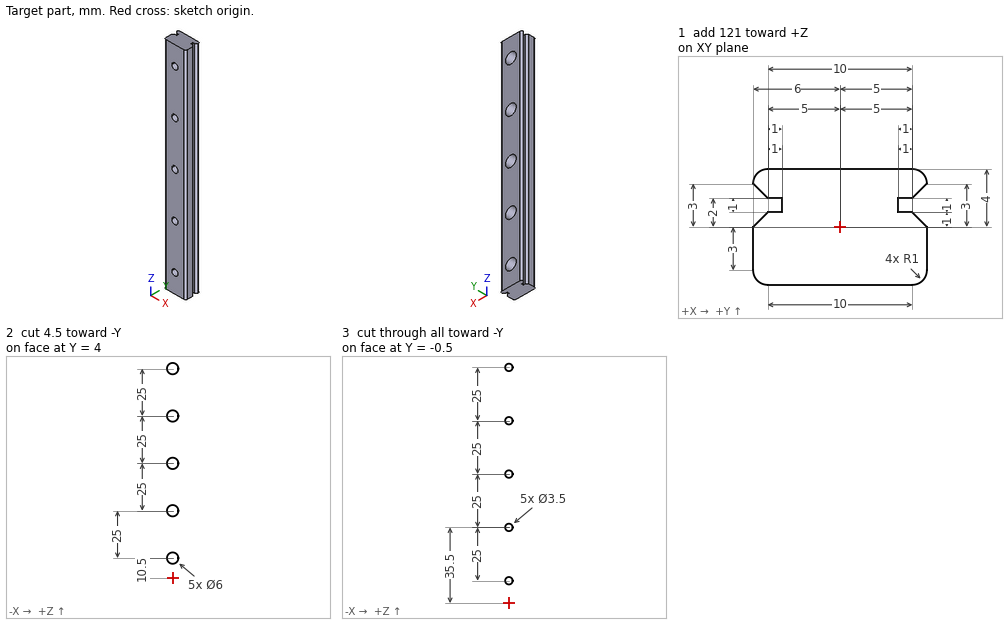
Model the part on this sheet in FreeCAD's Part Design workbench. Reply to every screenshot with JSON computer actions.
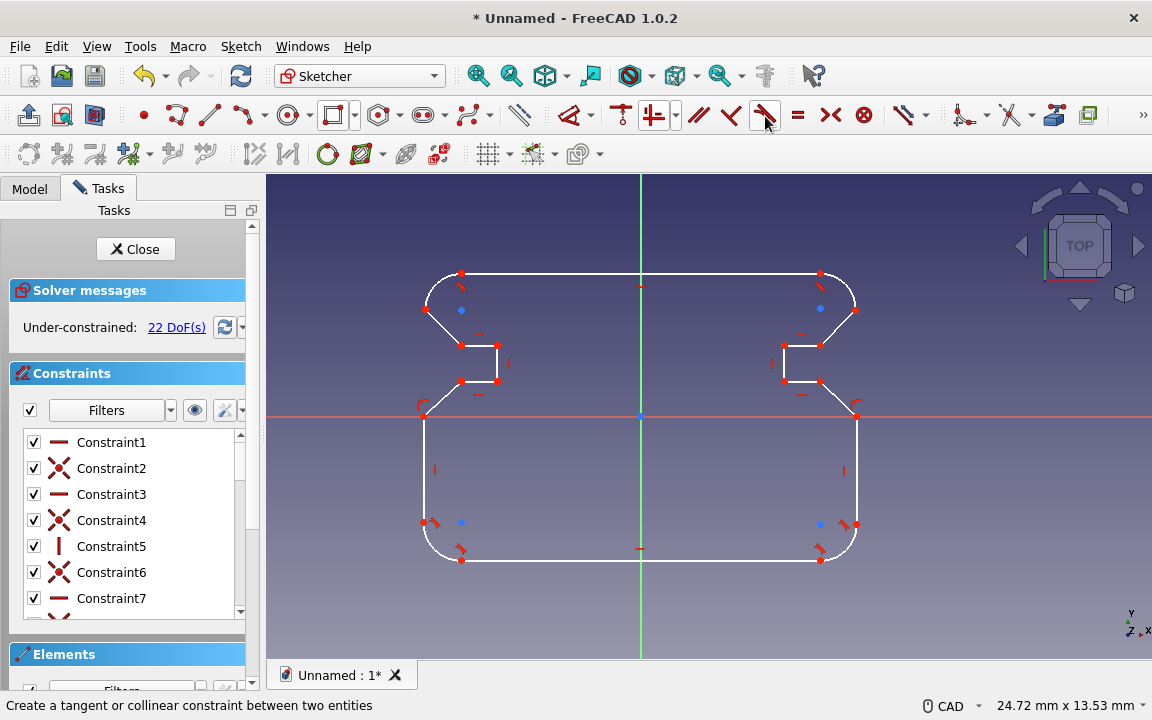
{"action": "left_click", "coordinate": [445, 278]}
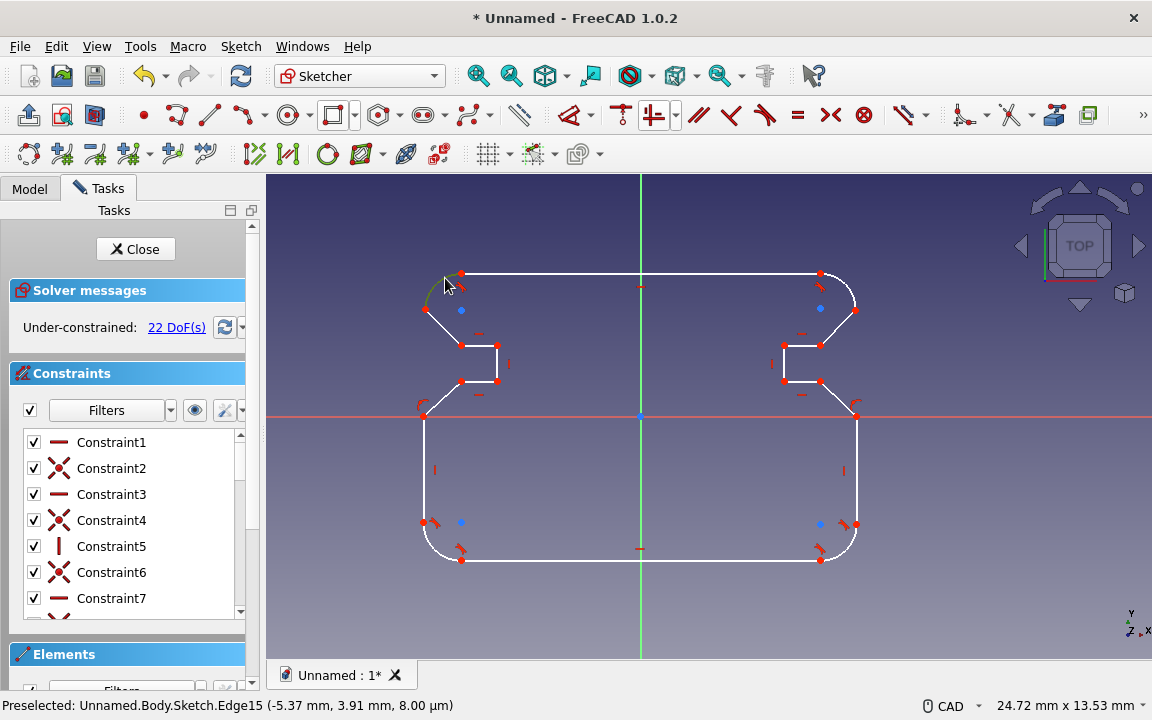
{"action": "left_click", "coordinate": [428, 540]}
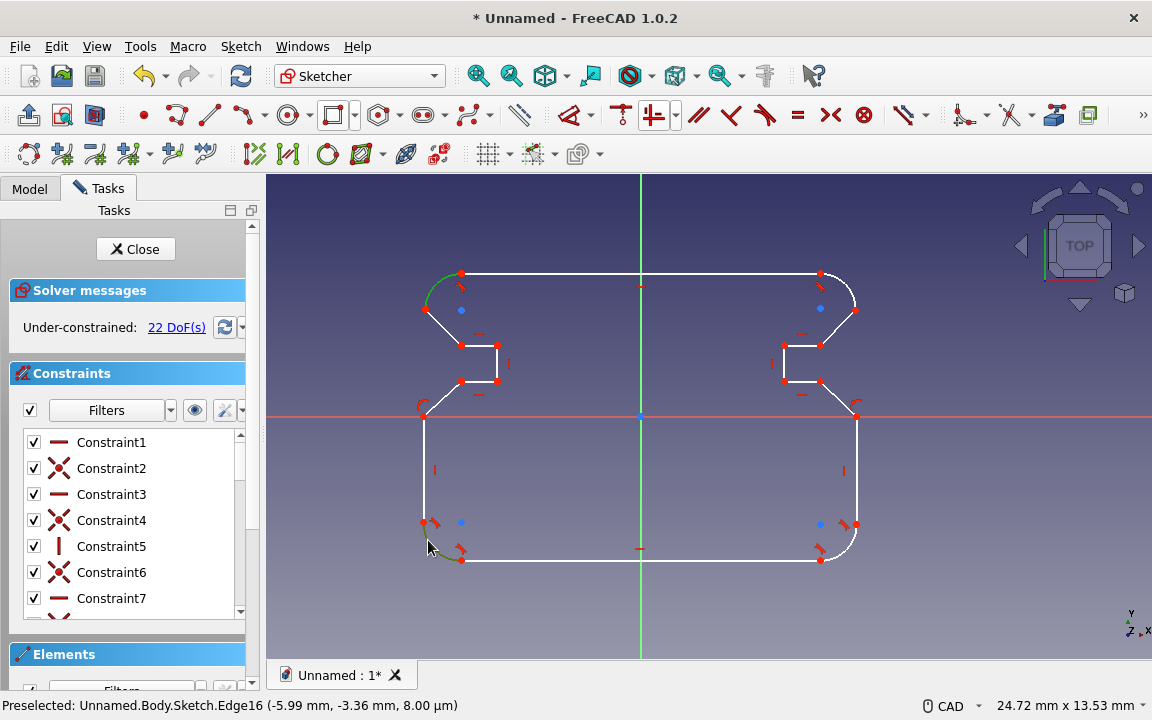
{"action": "left_click", "coordinate": [837, 557]}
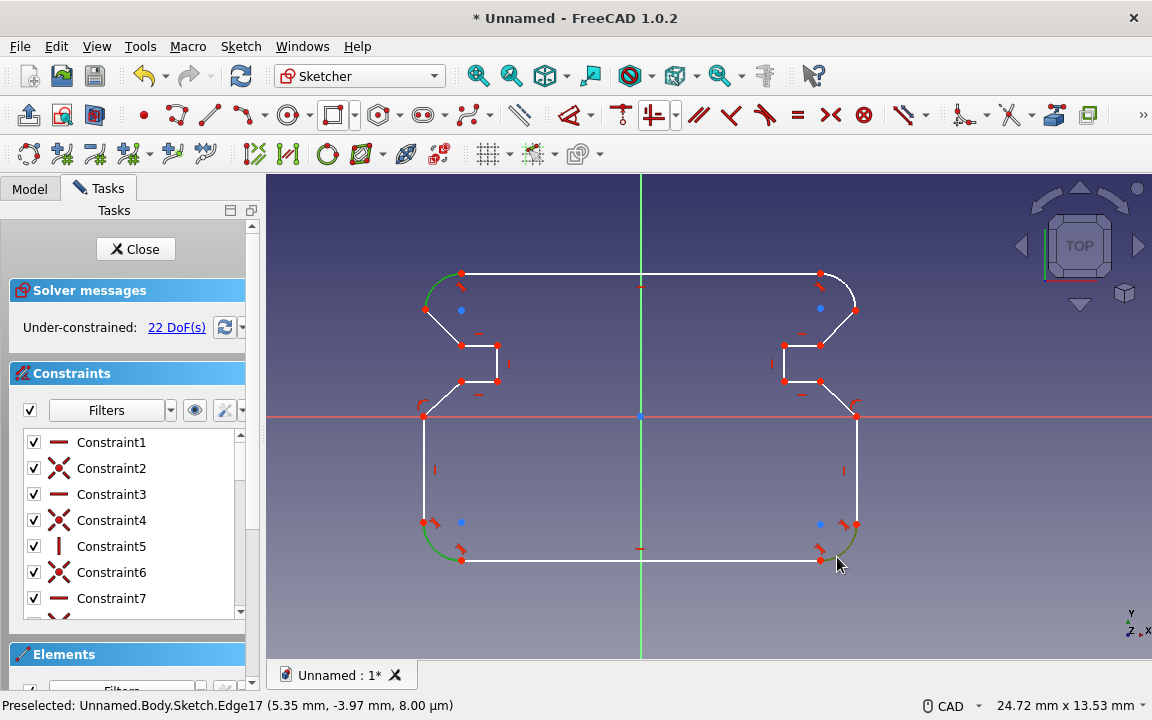
{"action": "left_click", "coordinate": [852, 294]}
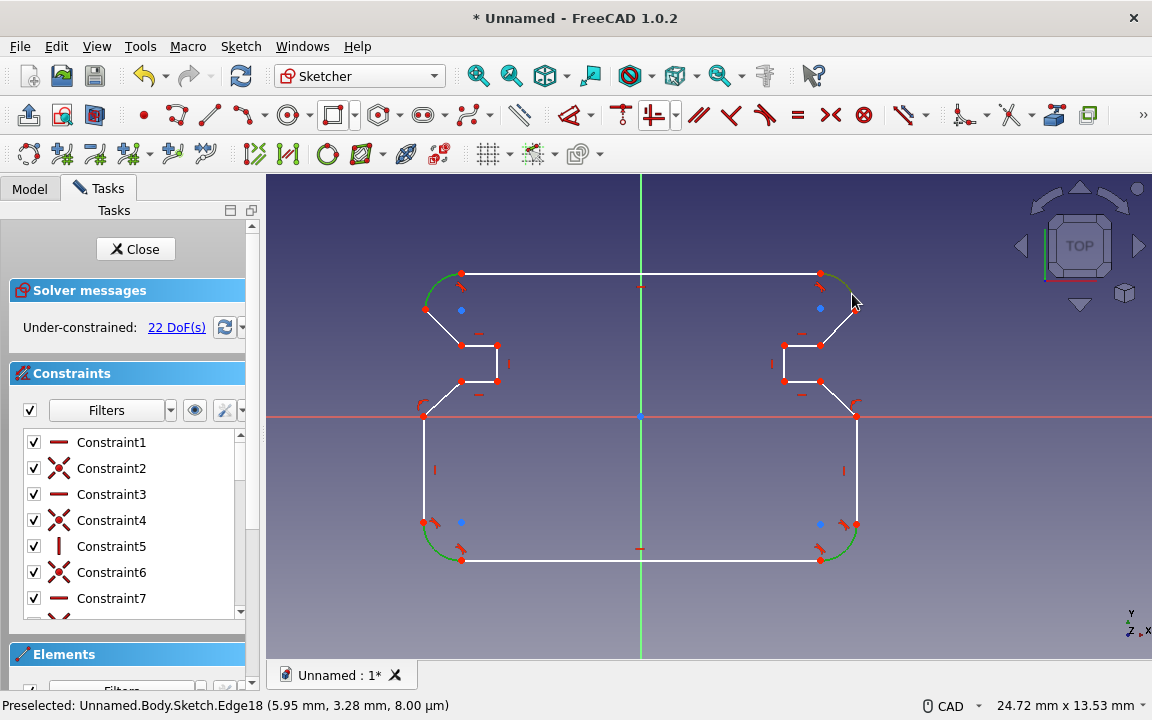
{"action": "left_click", "coordinate": [798, 116]}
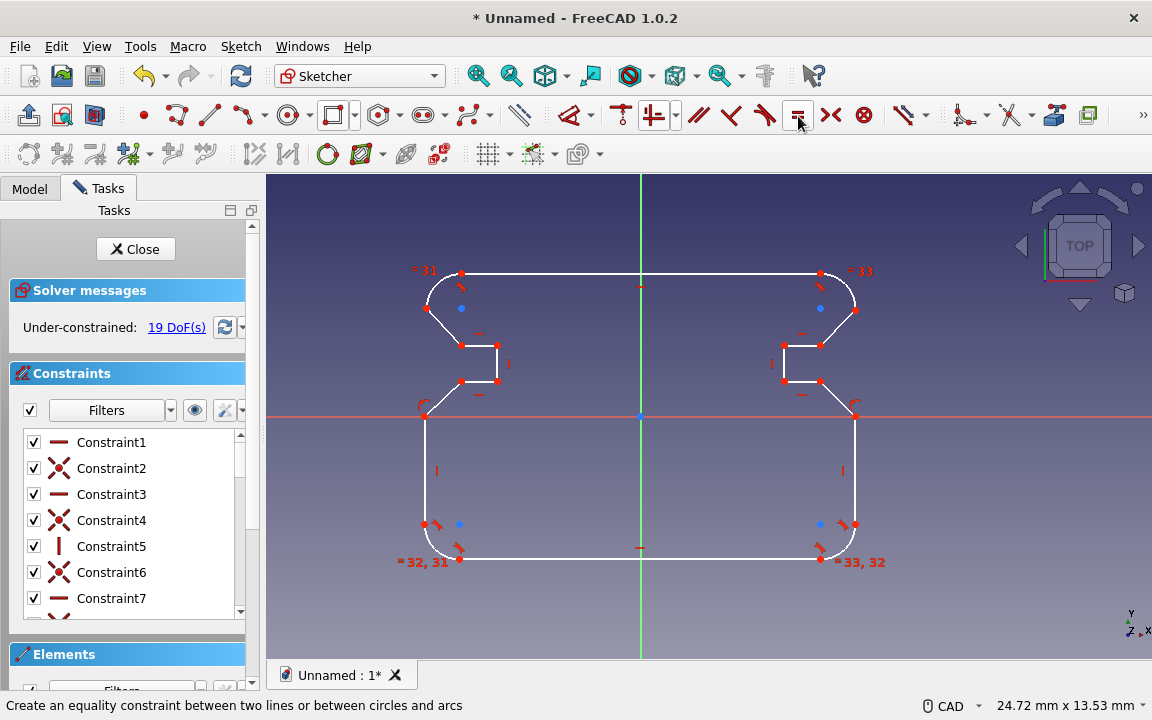
{"action": "left_click", "coordinate": [568, 116]}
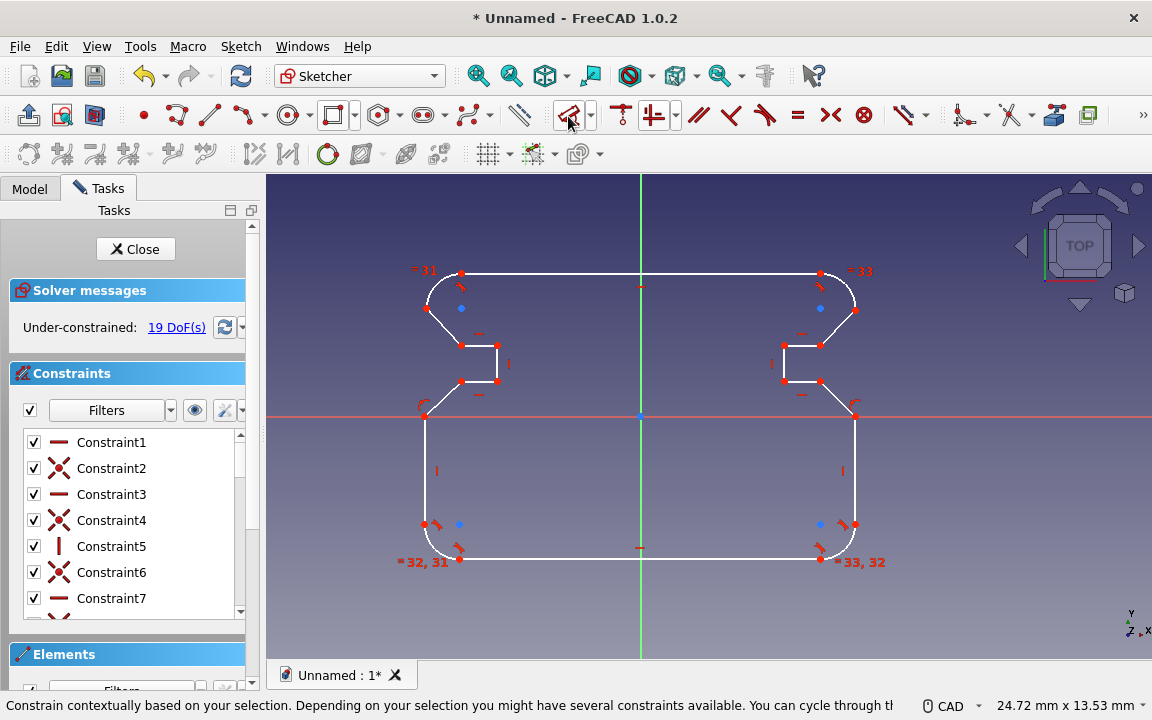
{"action": "left_click", "coordinate": [446, 278]}
{"action": "left_click", "coordinate": [432, 249]}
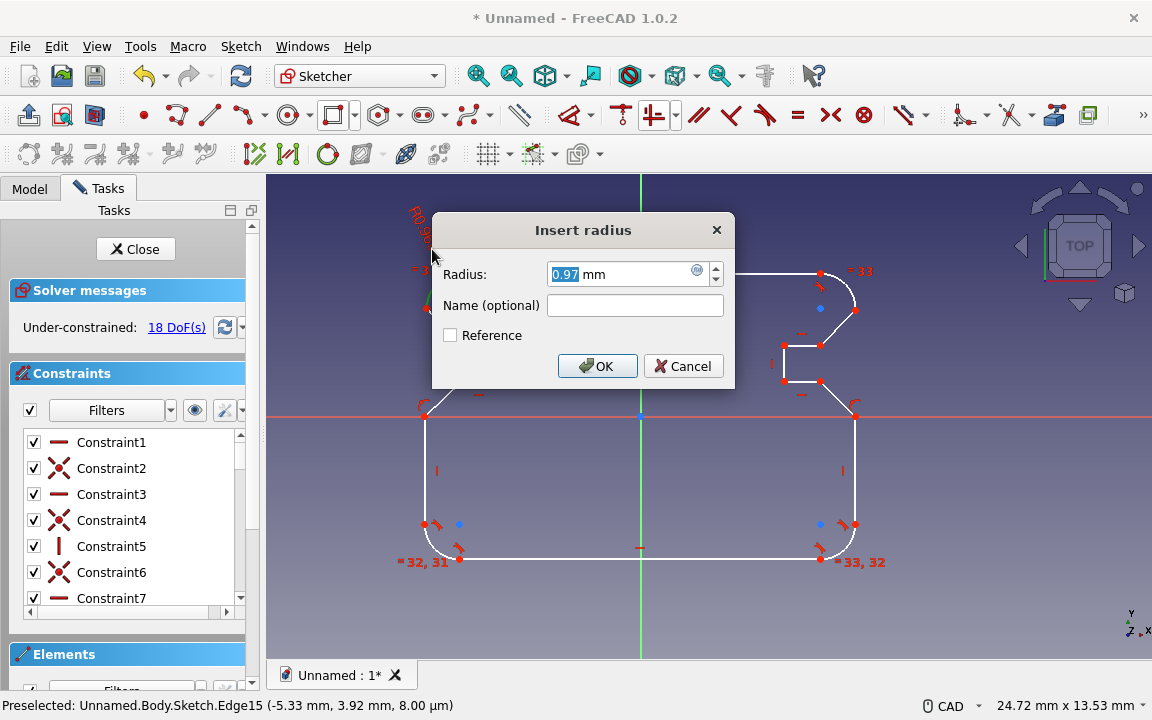
{"action": "type", "text": "1"}
{"action": "key", "text": "Return"}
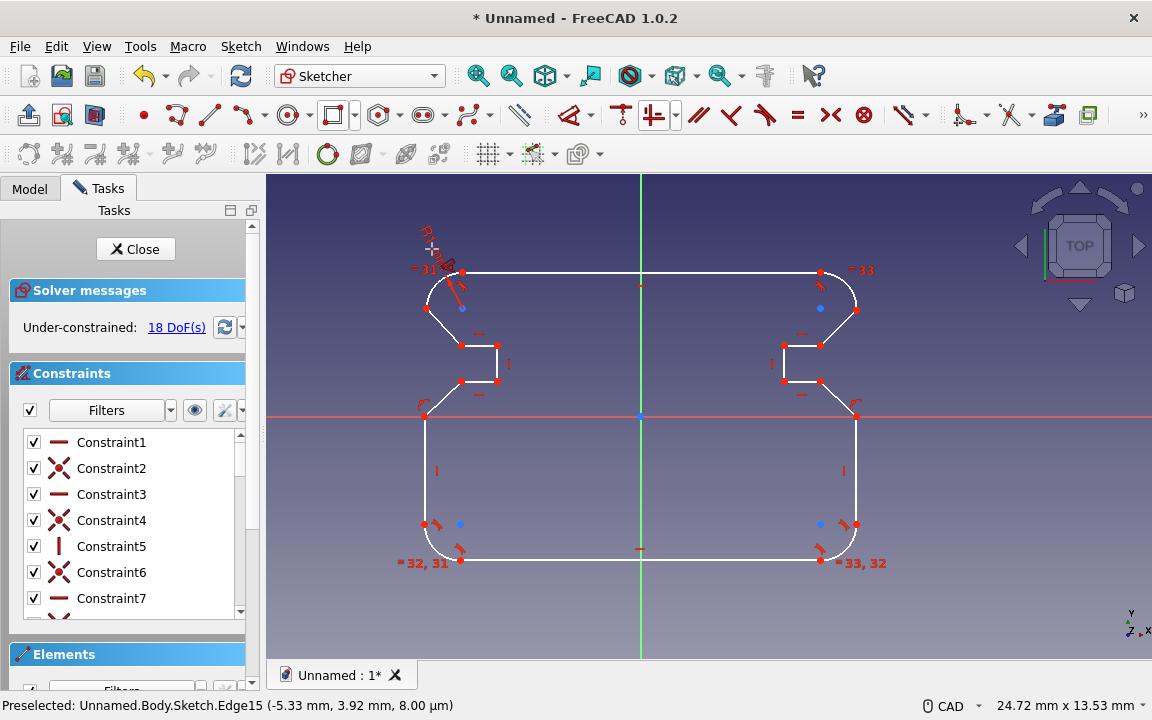
{"action": "scroll", "coordinate": [472, 346], "scroll_direction": "up", "scroll_amount": 2}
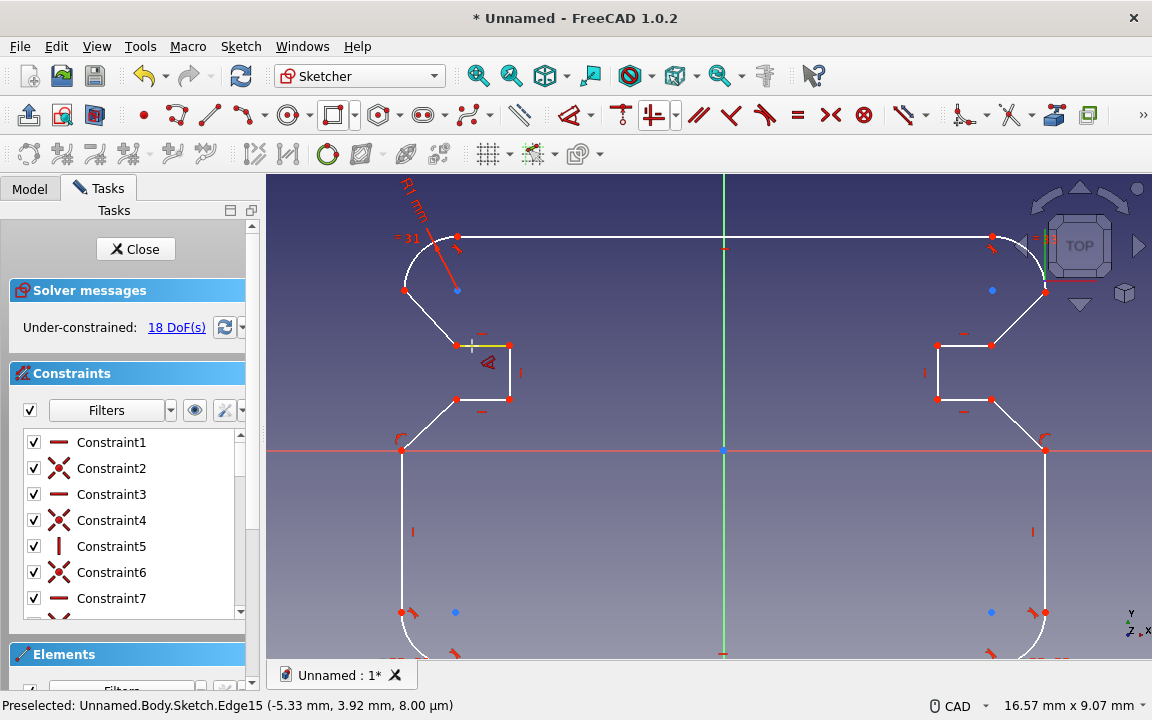
{"action": "left_click", "coordinate": [472, 346]}
{"action": "left_click", "coordinate": [483, 312]}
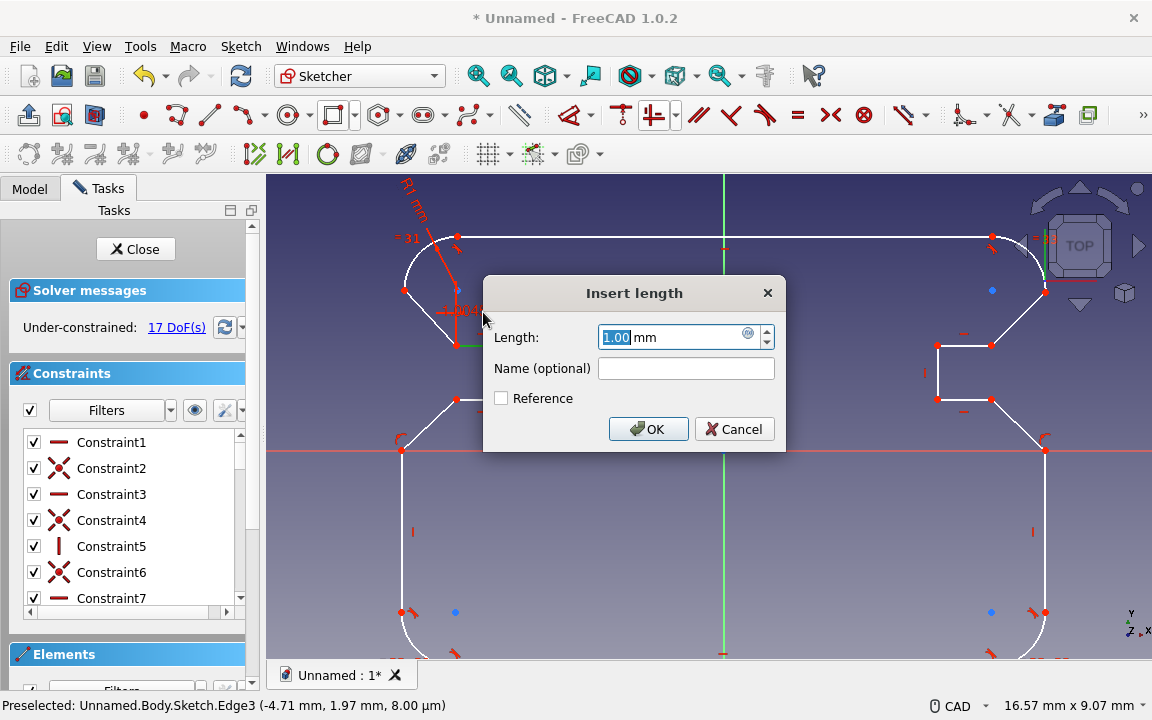
{"action": "type", "text": "1"}
{"action": "key", "text": "Return"}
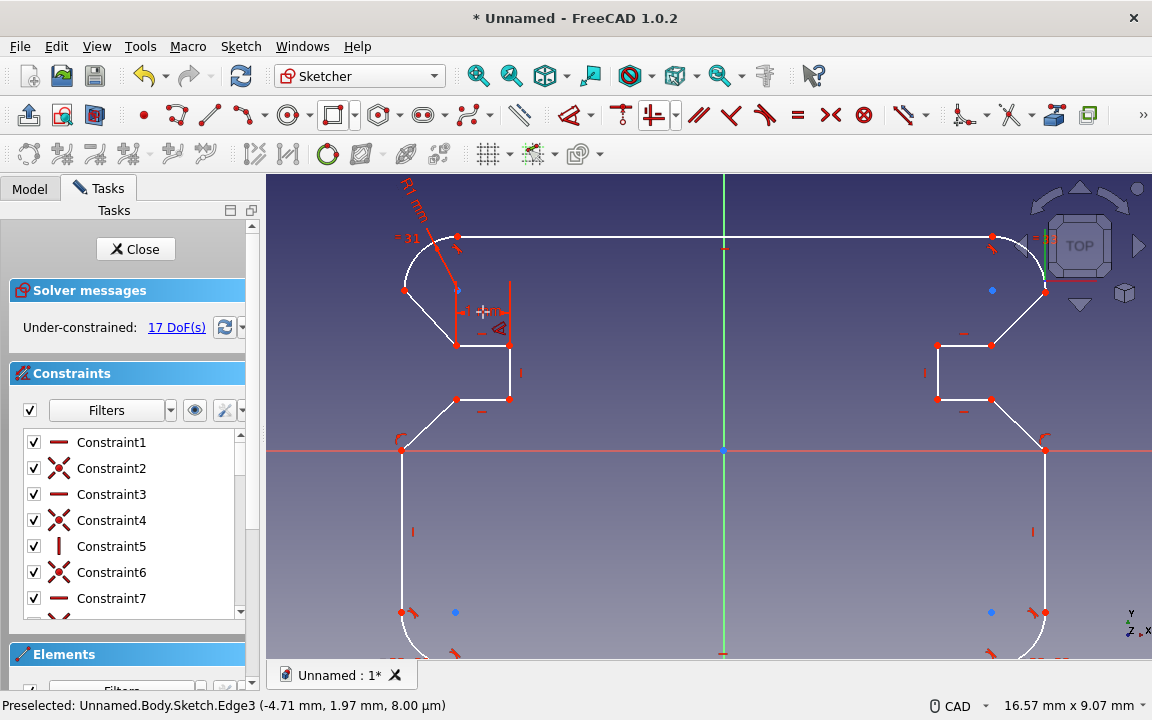
{"action": "left_click", "coordinate": [510, 362]}
{"action": "left_click", "coordinate": [476, 373]}